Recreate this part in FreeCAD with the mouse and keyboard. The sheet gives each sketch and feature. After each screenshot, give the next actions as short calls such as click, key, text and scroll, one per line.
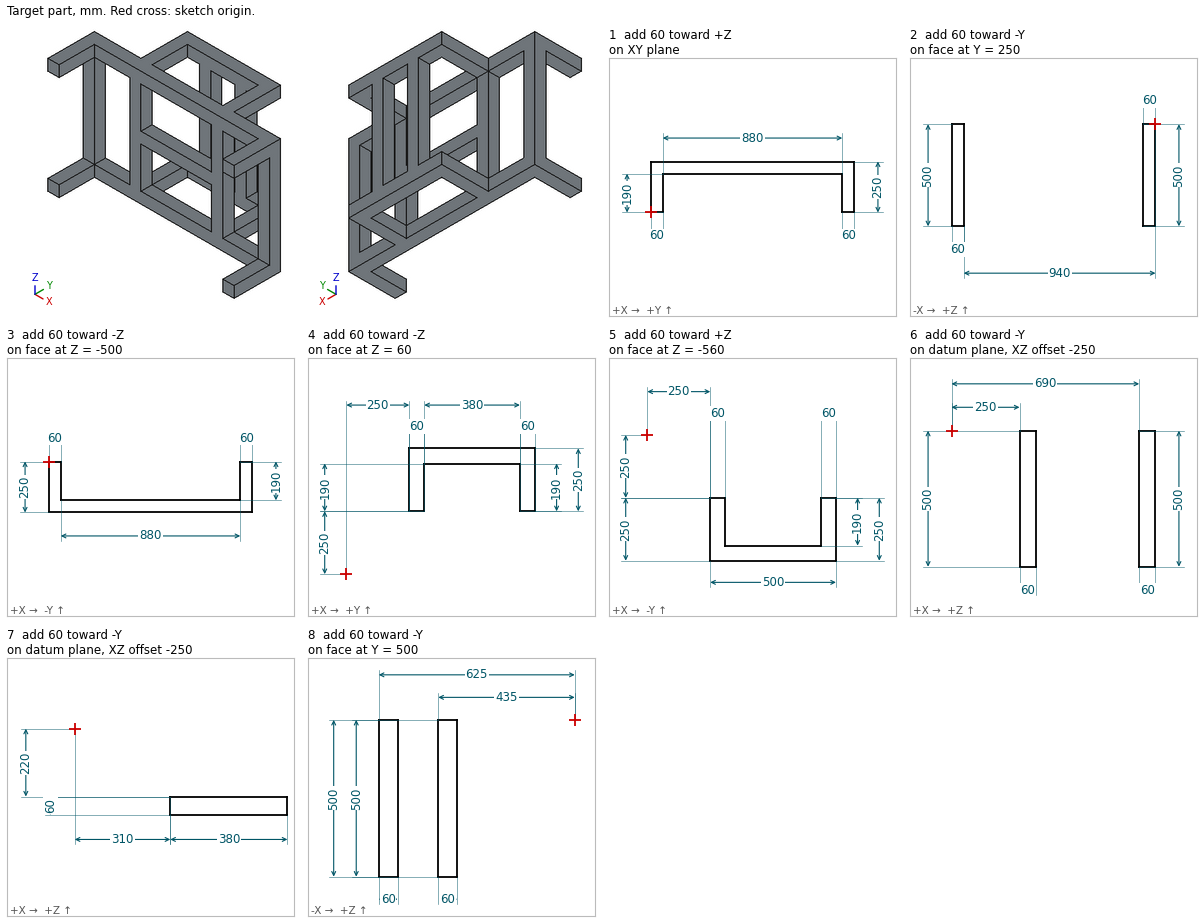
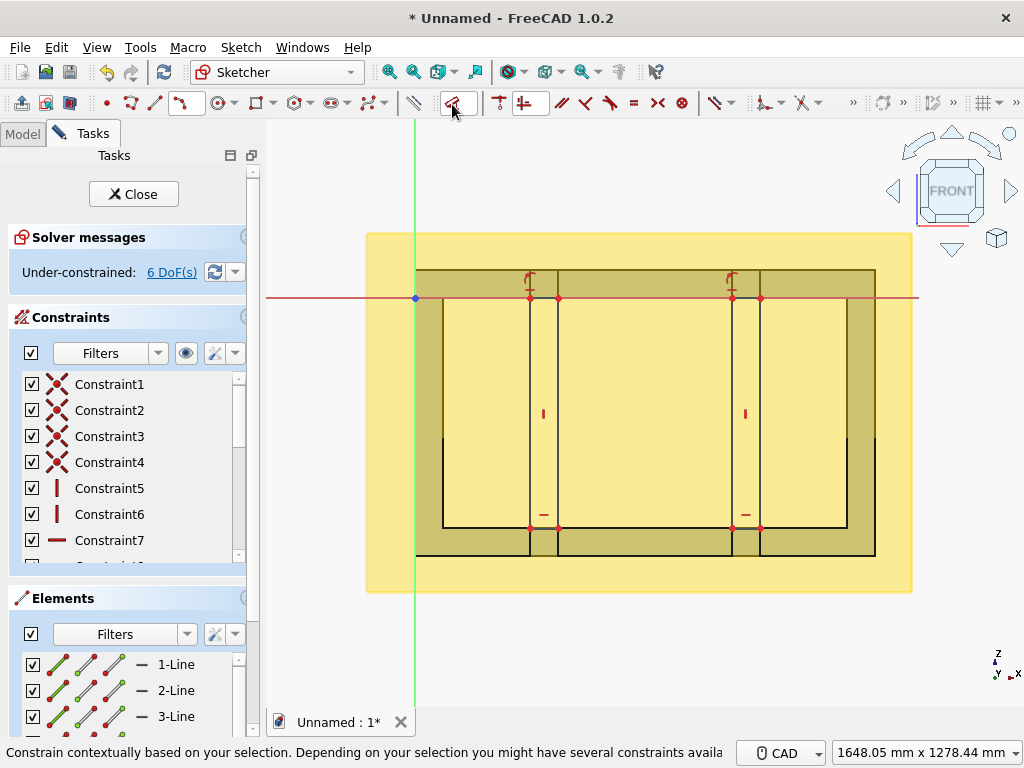
scroll(541, 529, up, 2)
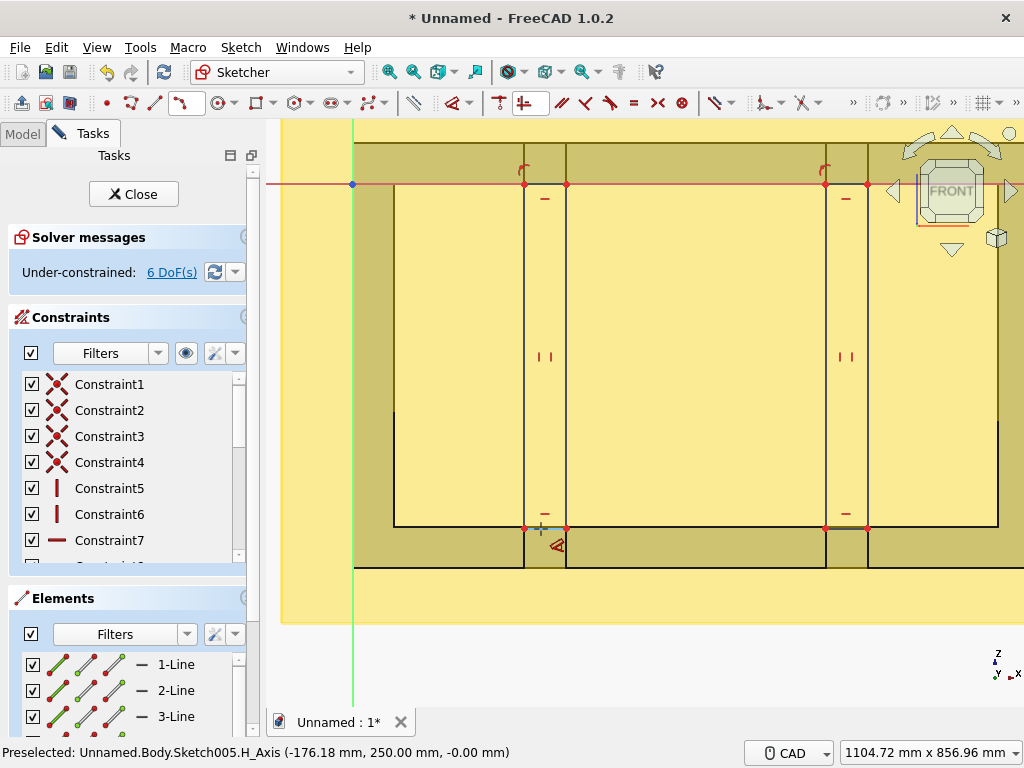
click(541, 529)
click(545, 563)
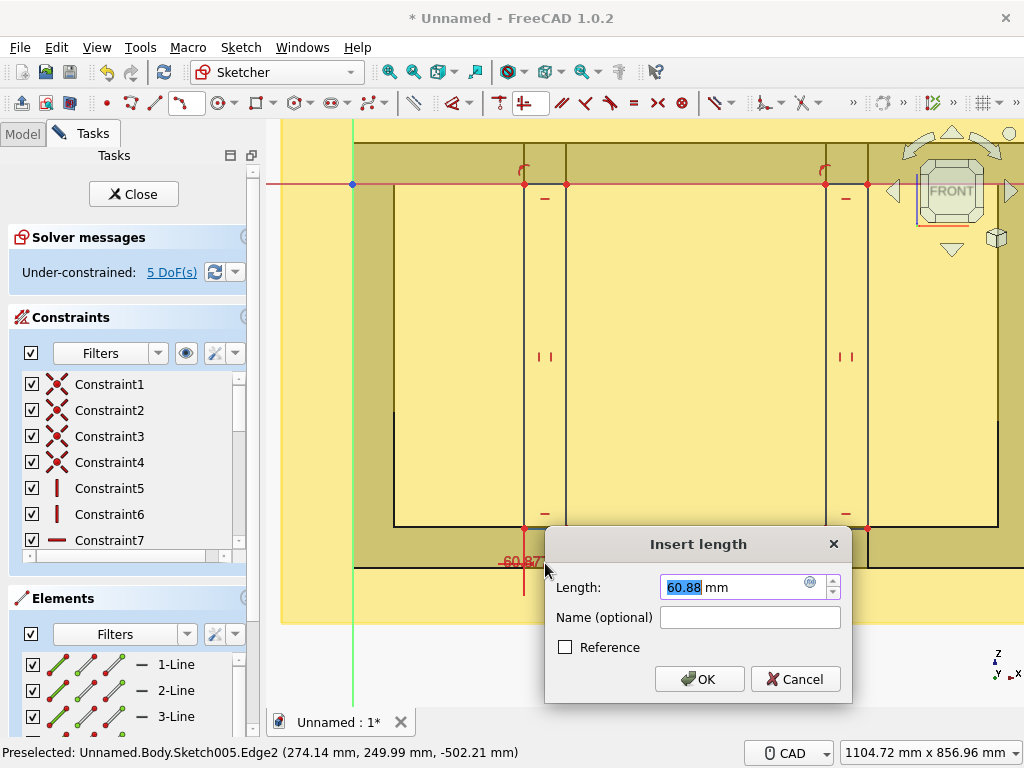
text(60)
key(Return)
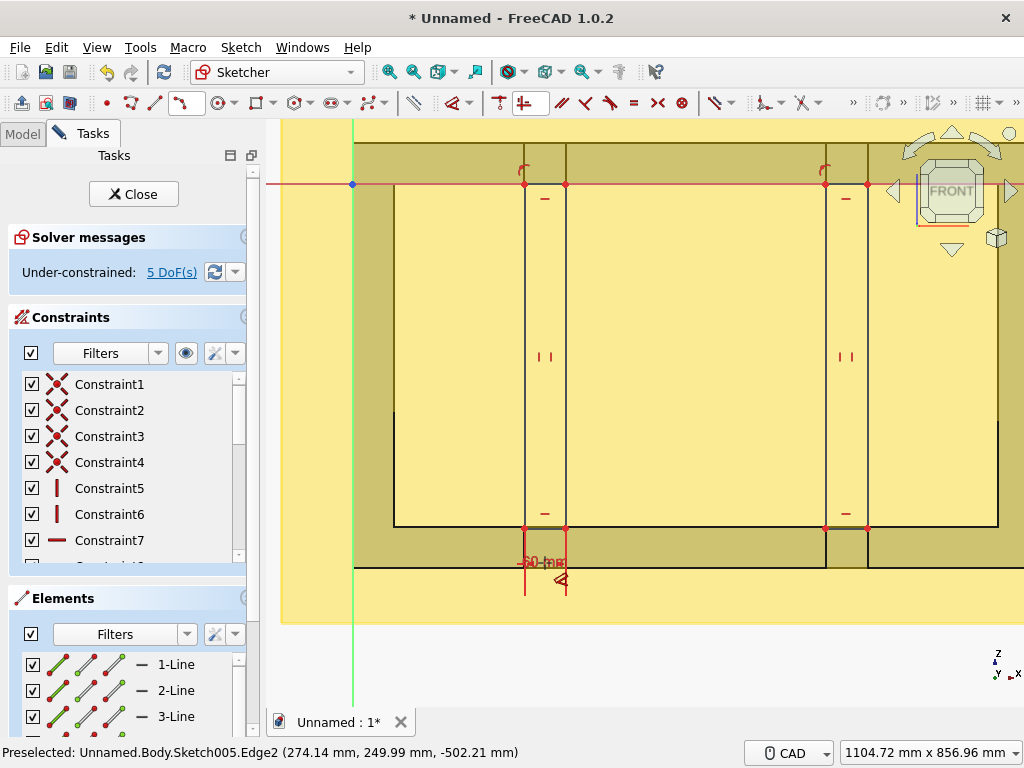
click(838, 529)
click(842, 563)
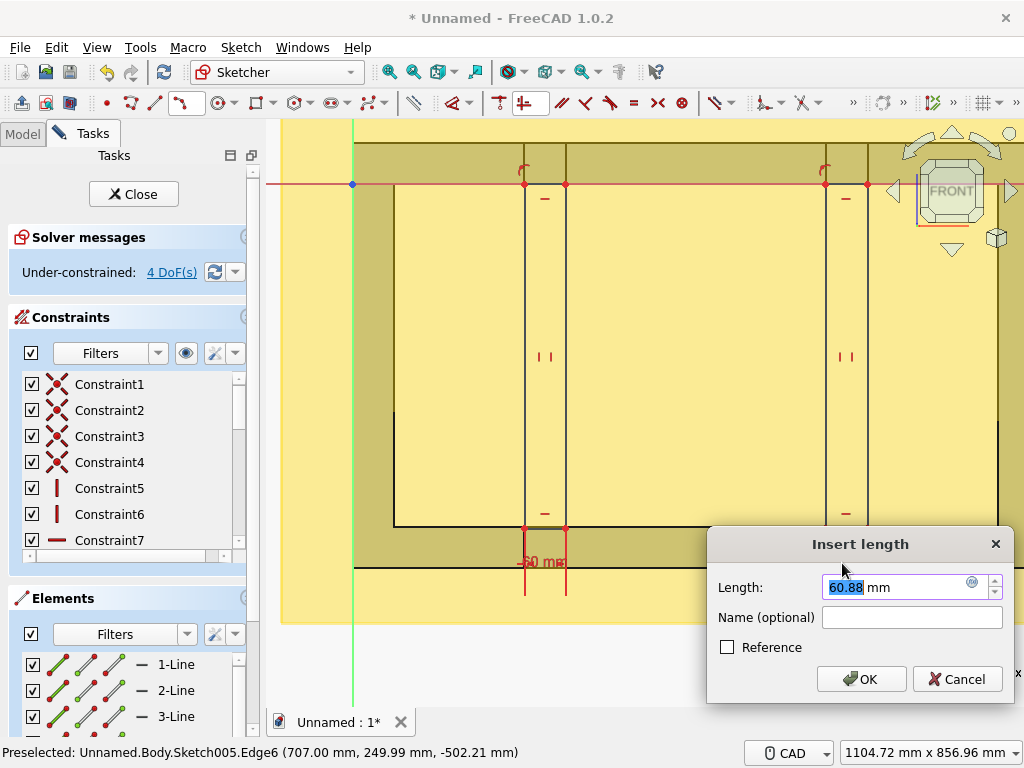
text(60)
key(Return)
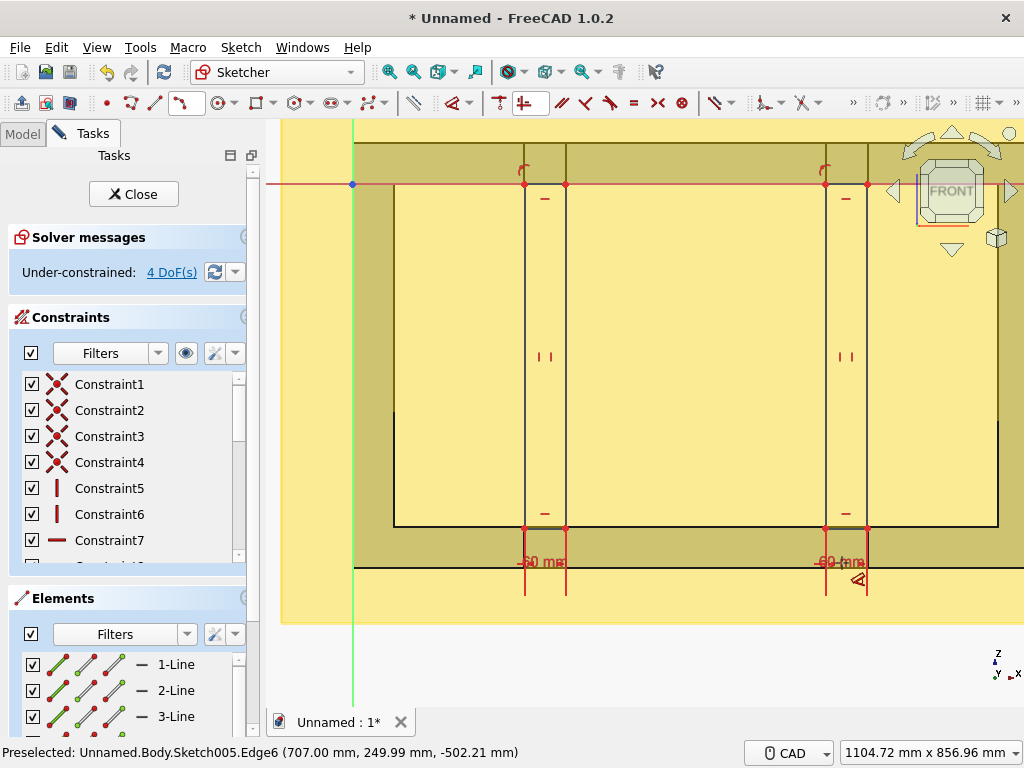
click(525, 287)
click(491, 356)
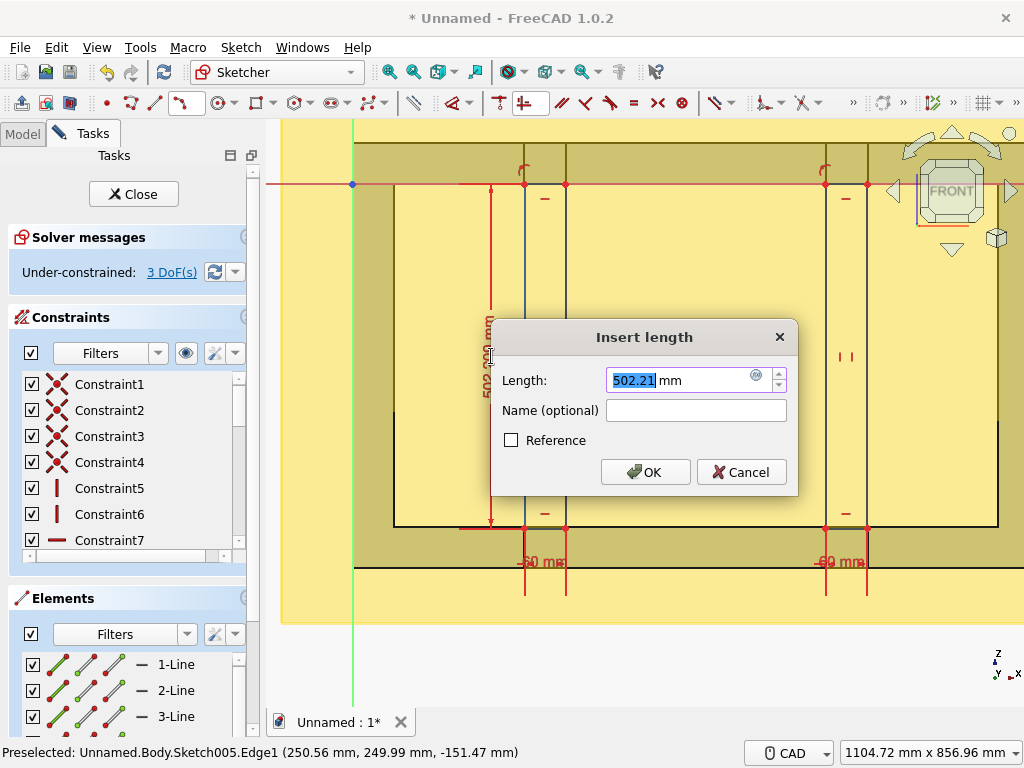
text(500)
key(Return)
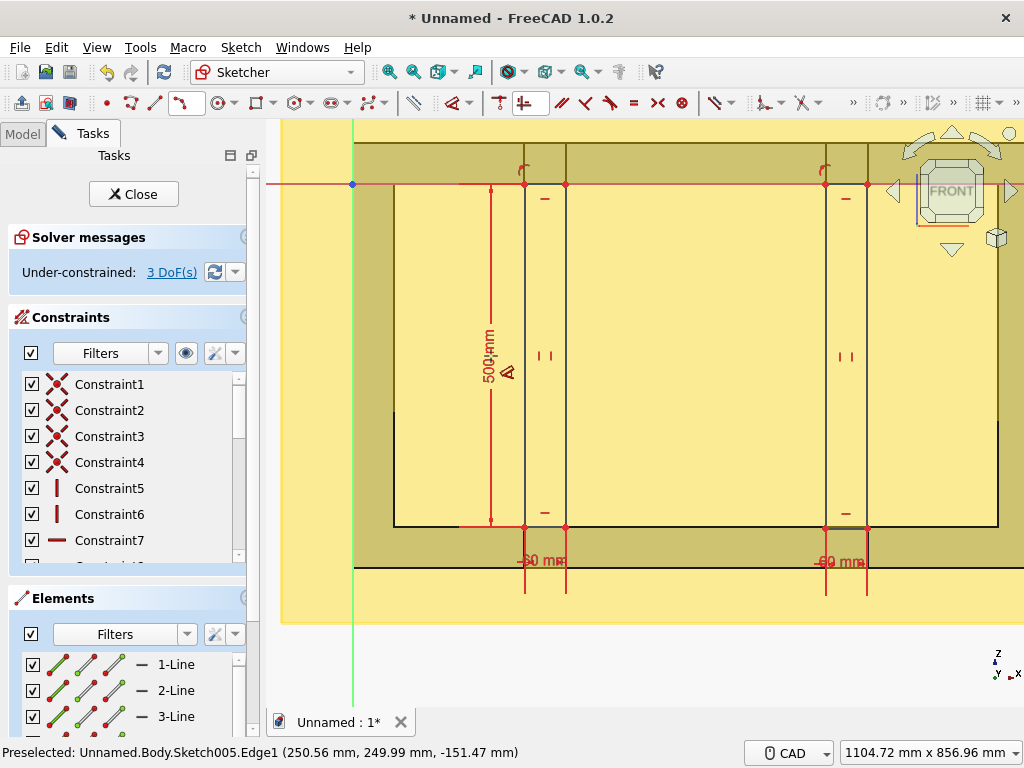
click(826, 287)
click(792, 356)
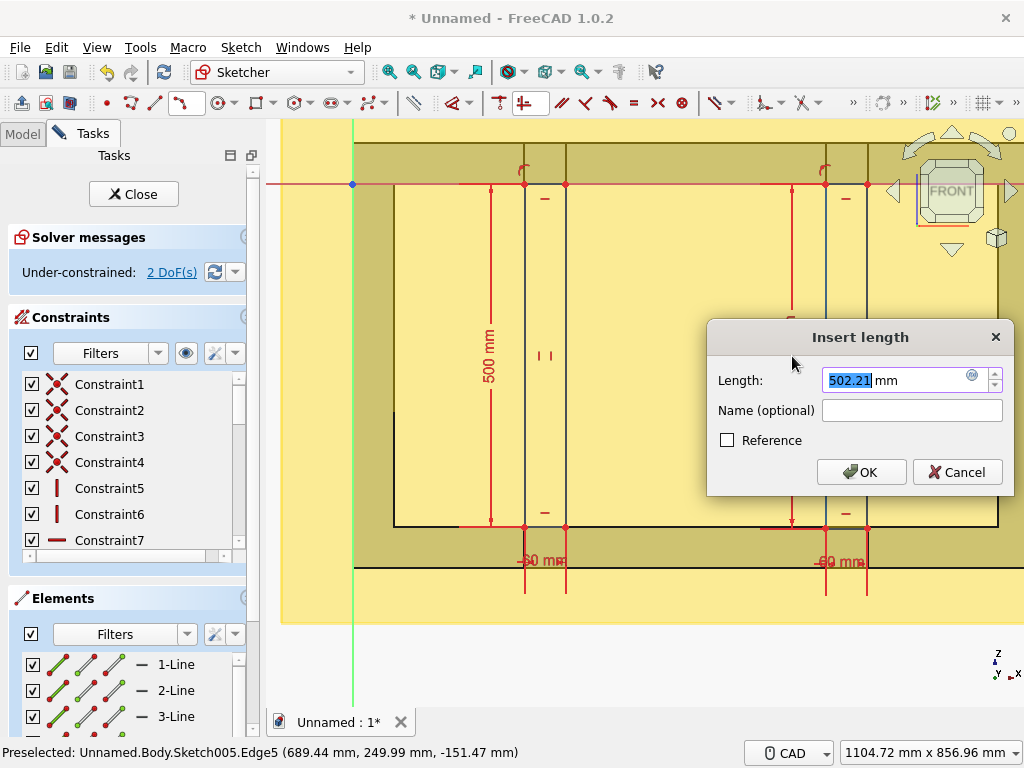
text(500)
key(Return)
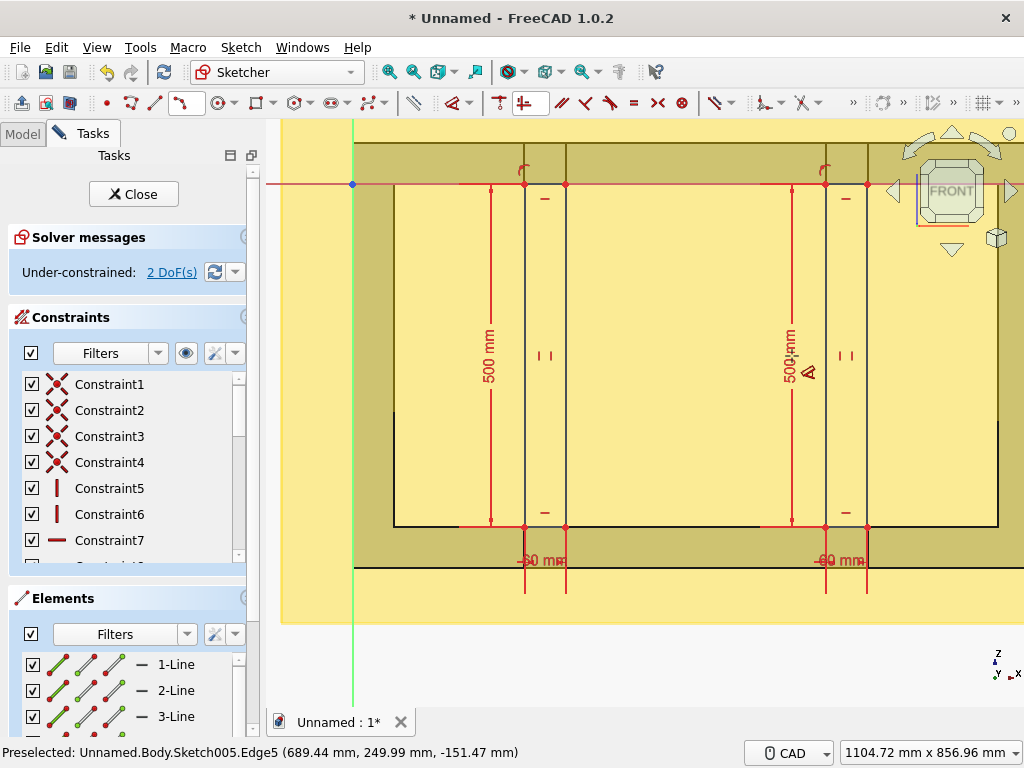
click(525, 184)
click(439, 150)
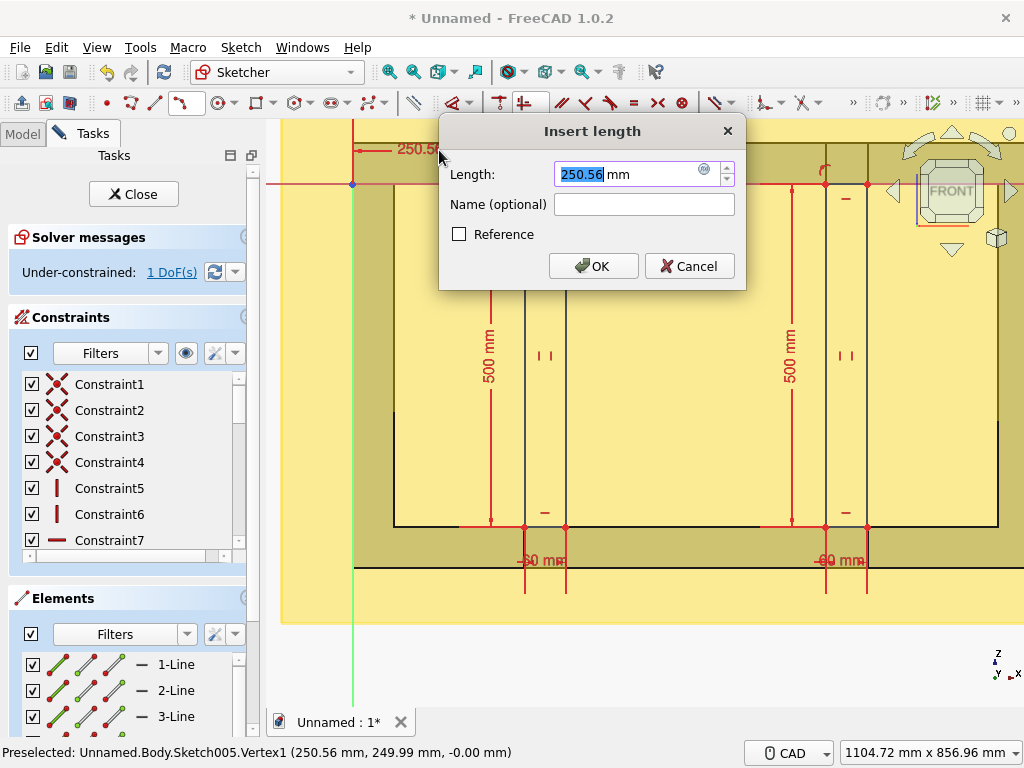
text(250)
key(Return)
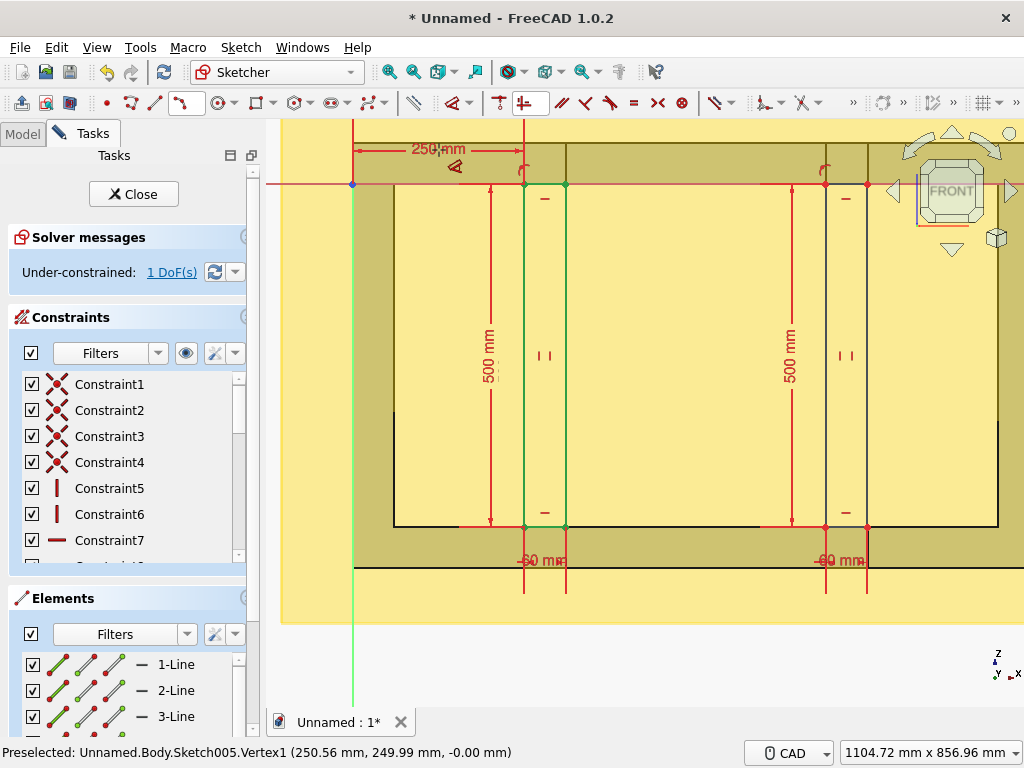
click(826, 184)
click(589, 150)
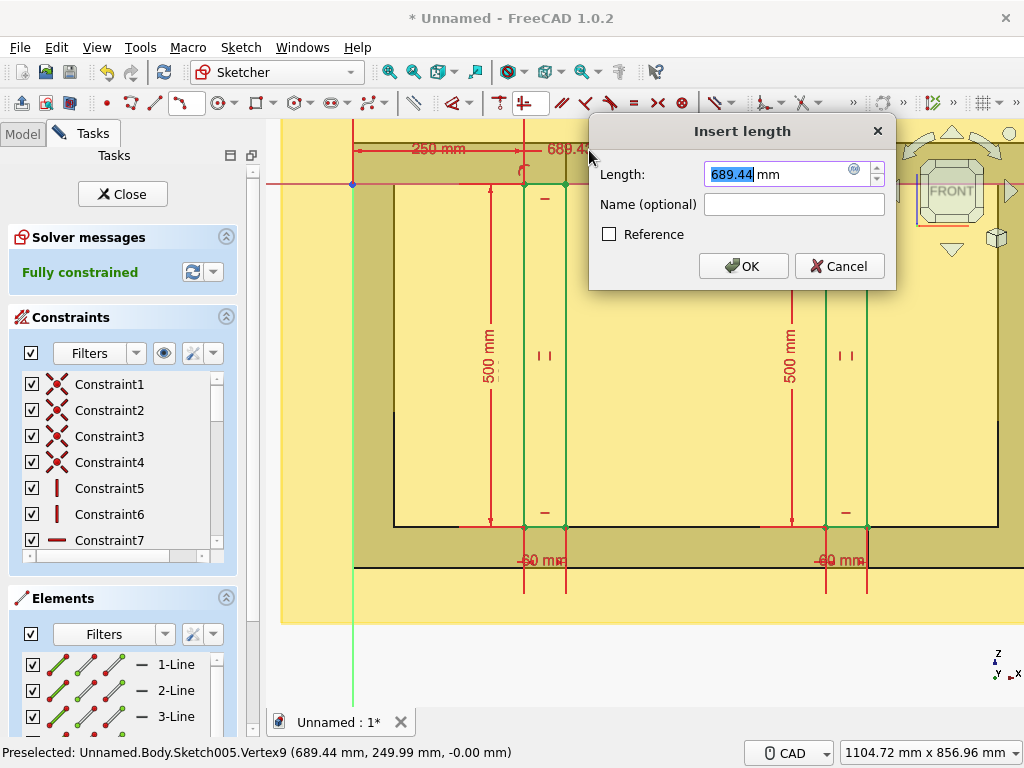
text(690)
key(Return)
key(Escape)